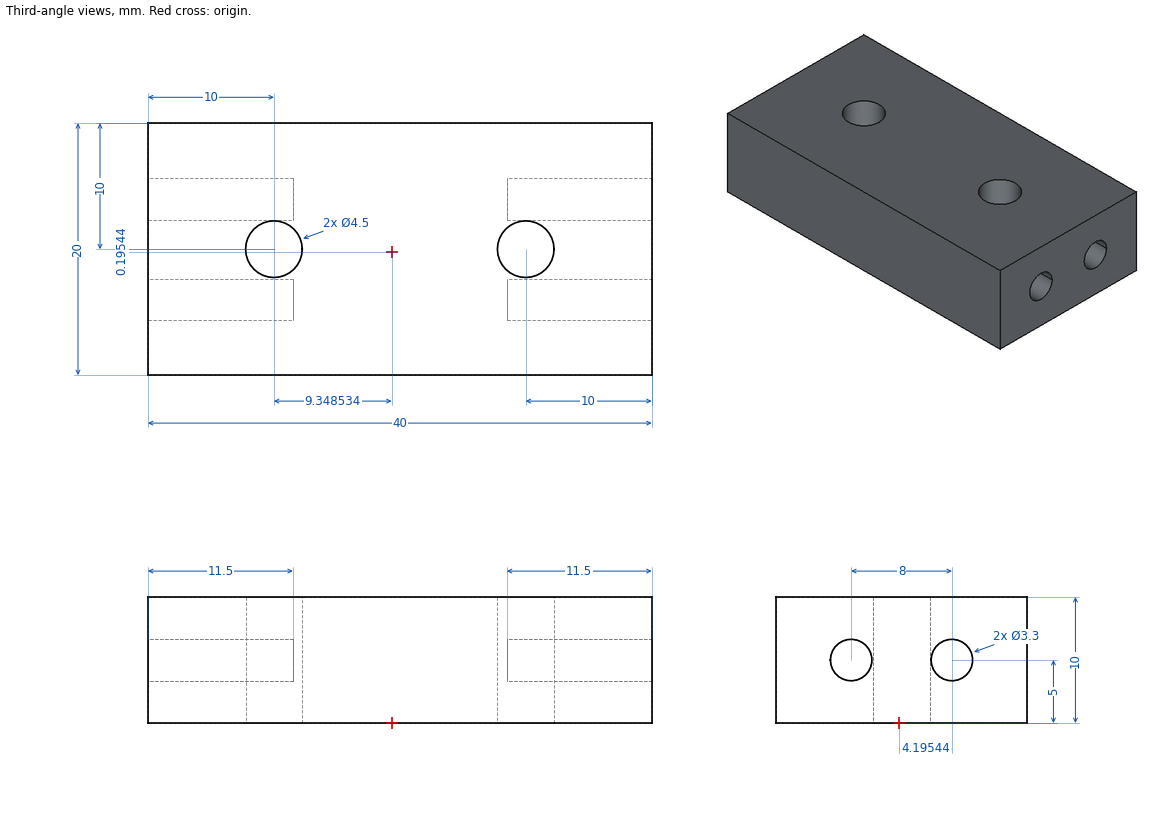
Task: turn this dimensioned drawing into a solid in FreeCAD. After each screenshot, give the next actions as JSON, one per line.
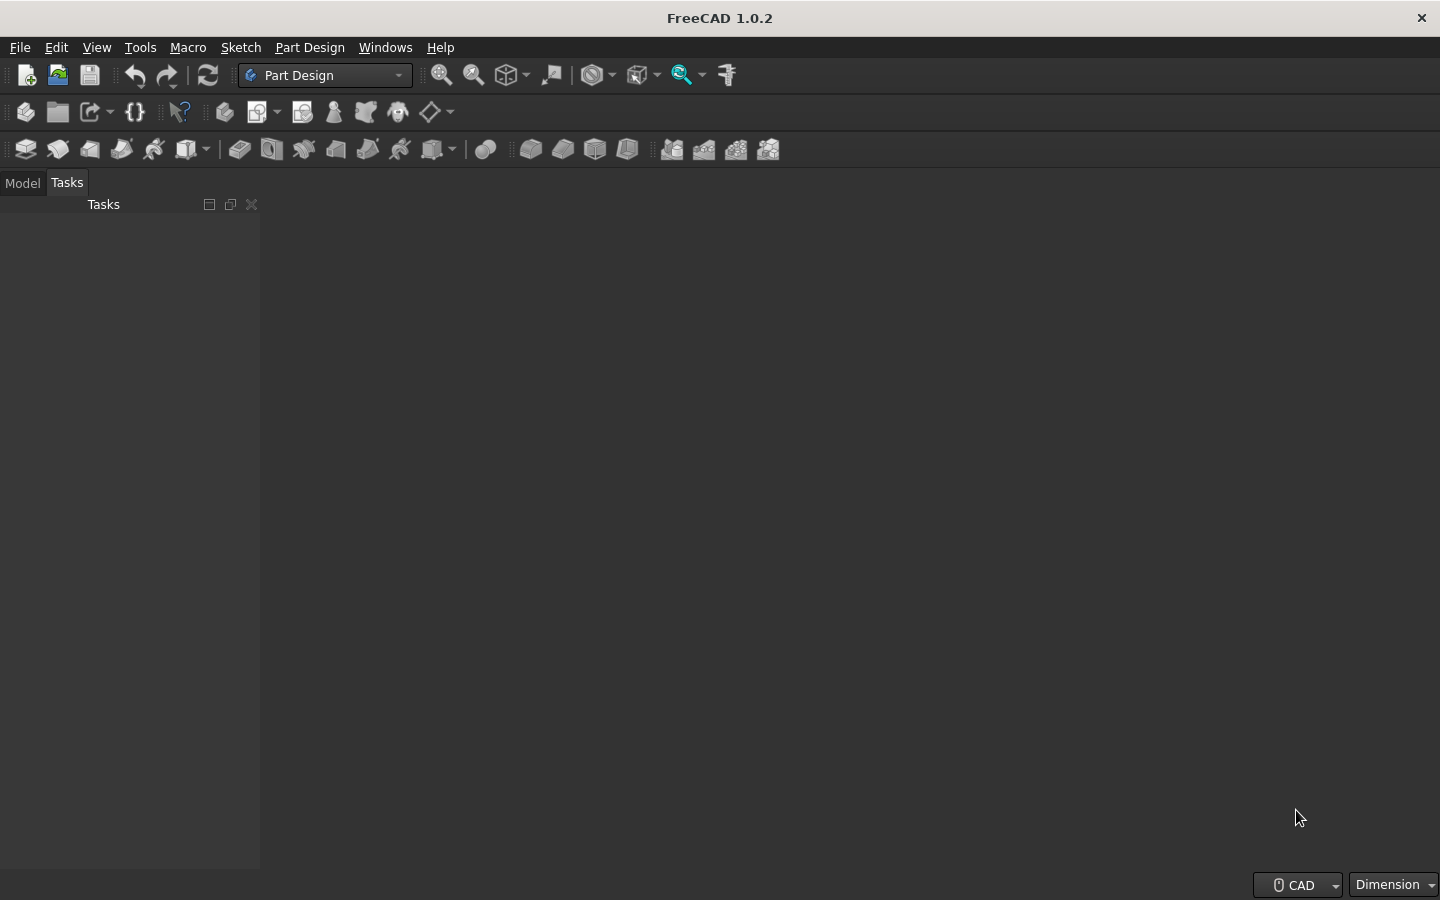
{"action": "left_click", "coordinate": [26, 76]}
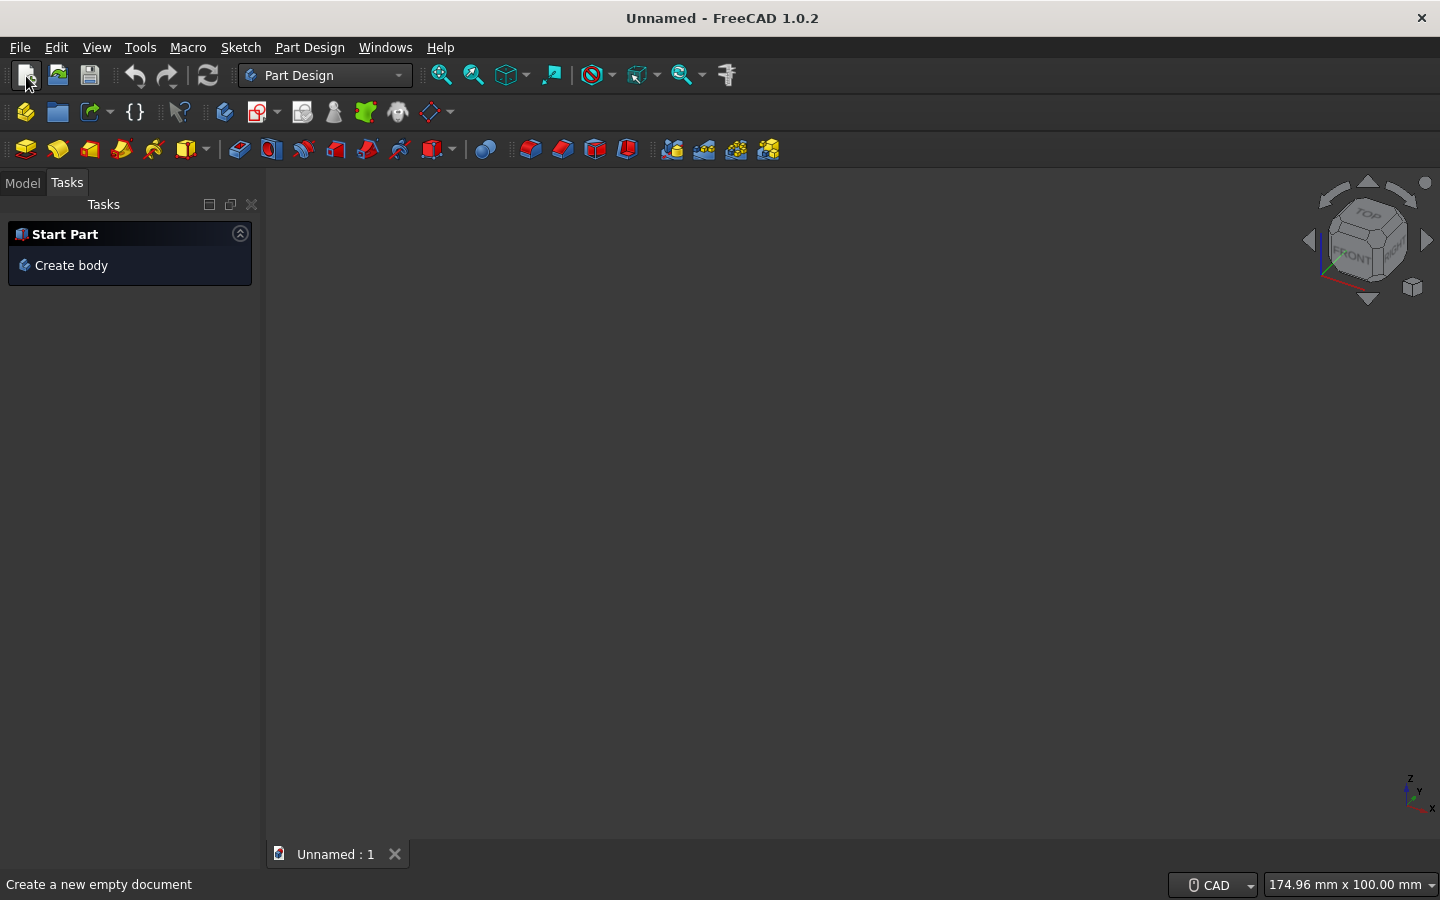
{"action": "left_click", "coordinate": [258, 112]}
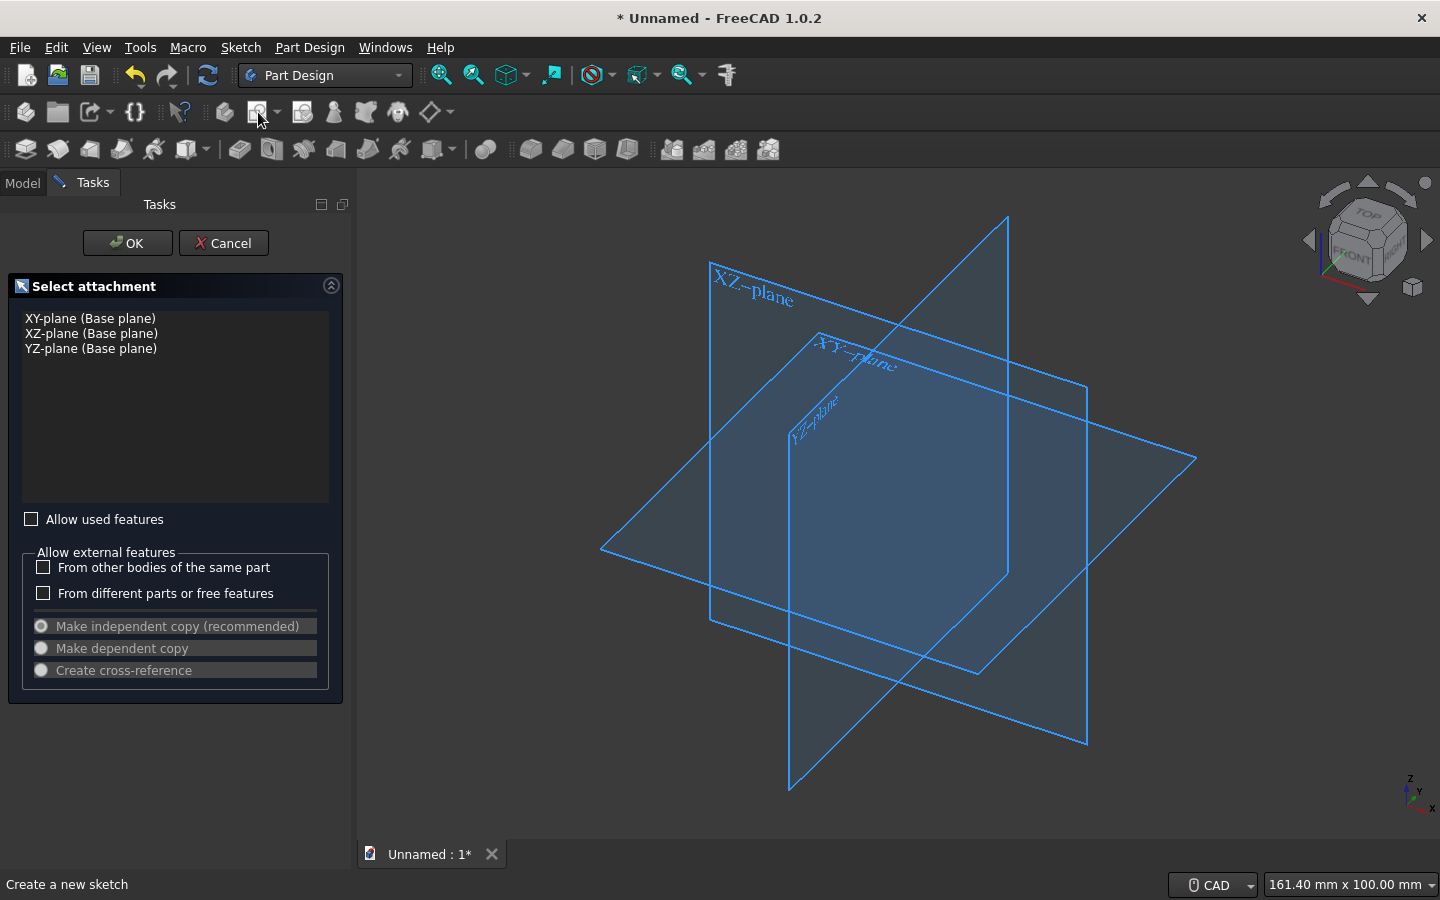
{"action": "left_click", "coordinate": [82, 318]}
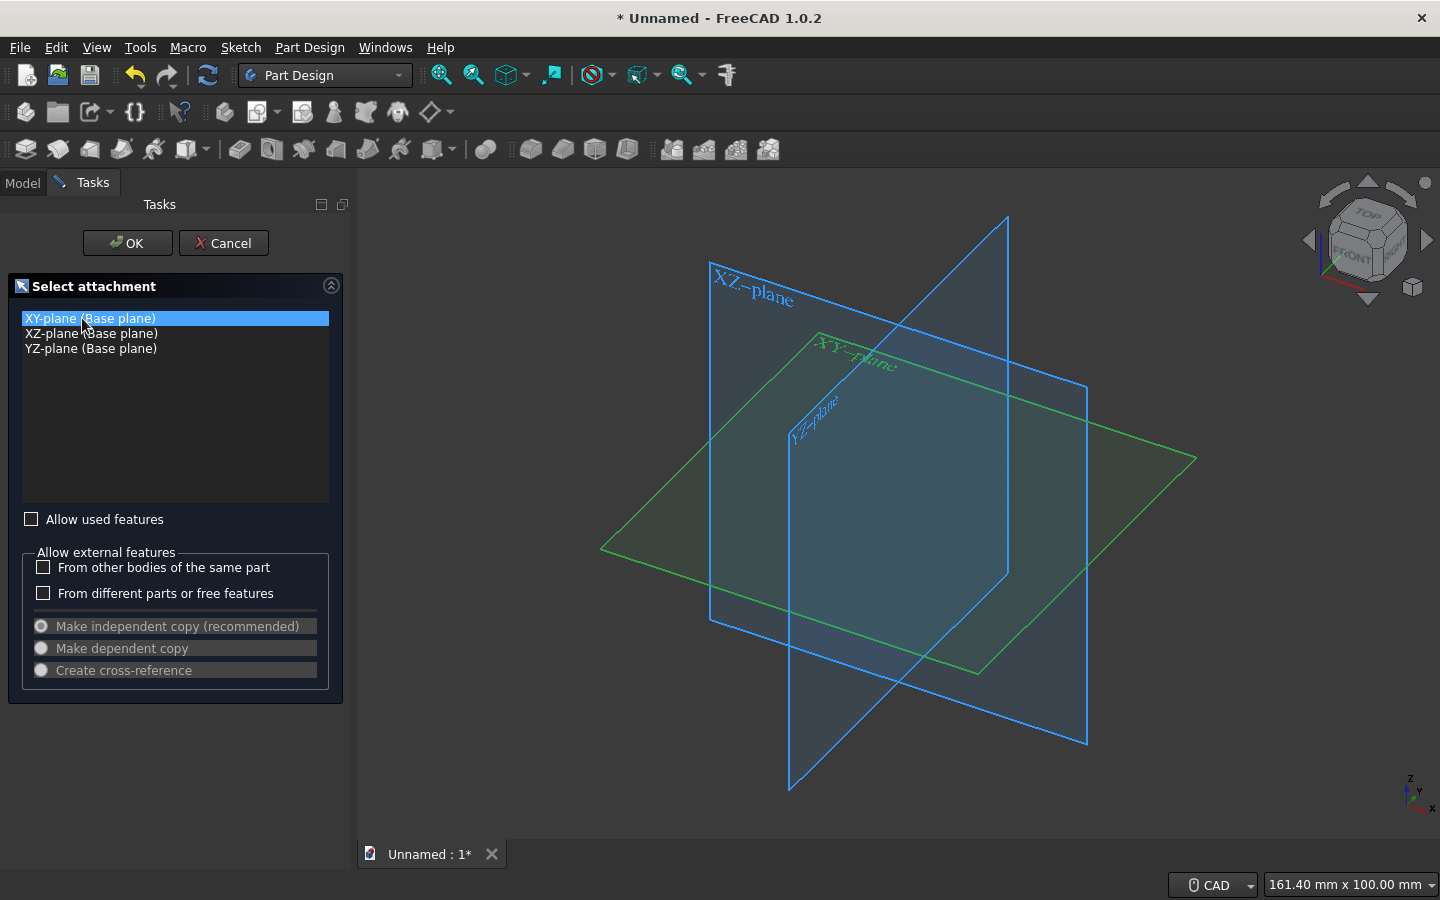
{"action": "left_click", "coordinate": [128, 243]}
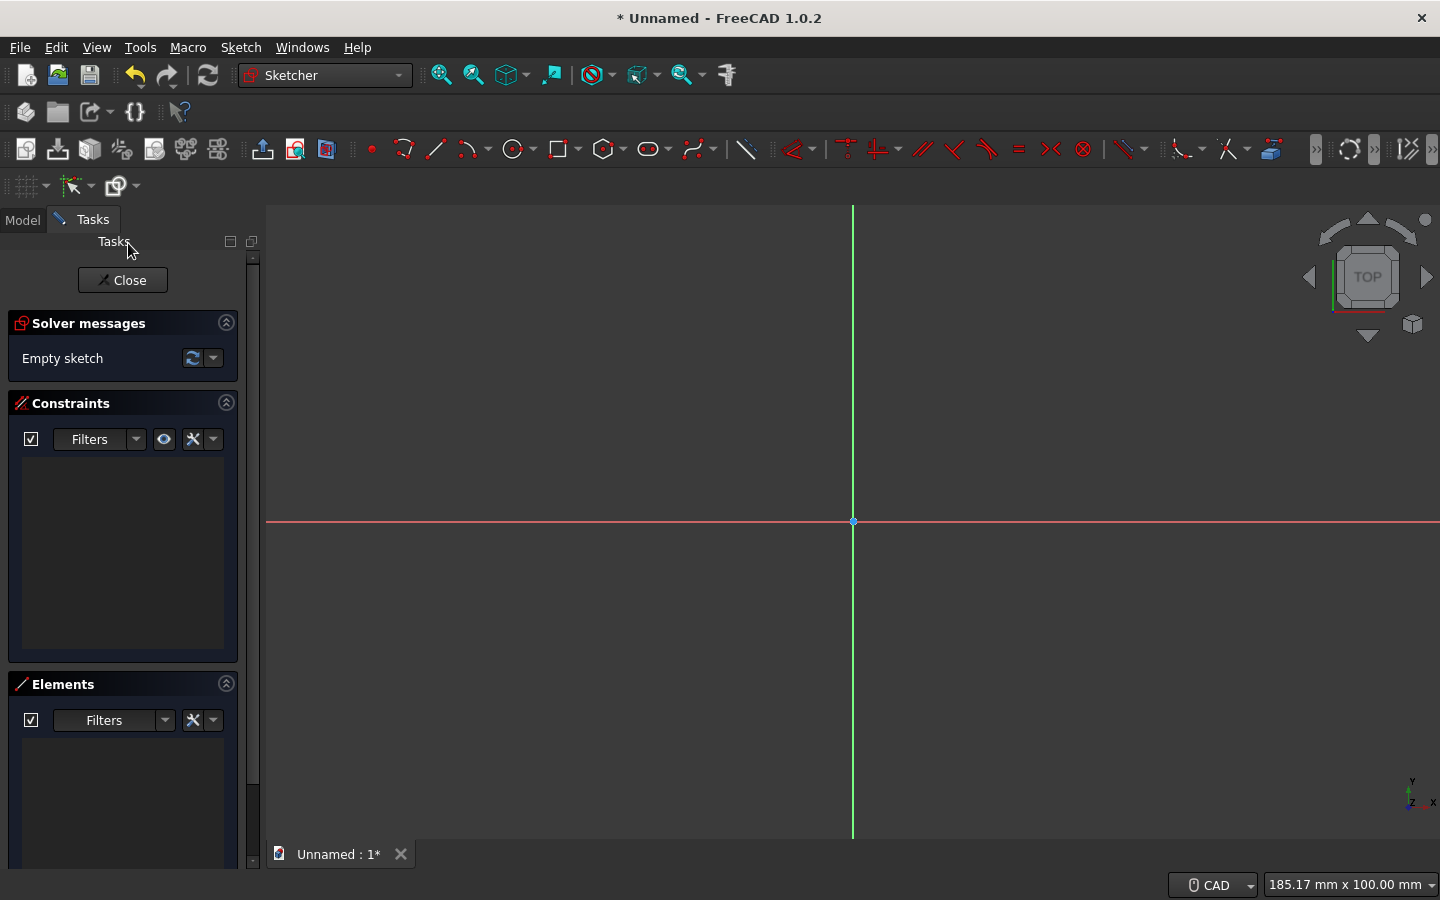
{"action": "scroll", "coordinate": [899, 520], "scroll_direction": "up", "scroll_amount": 5}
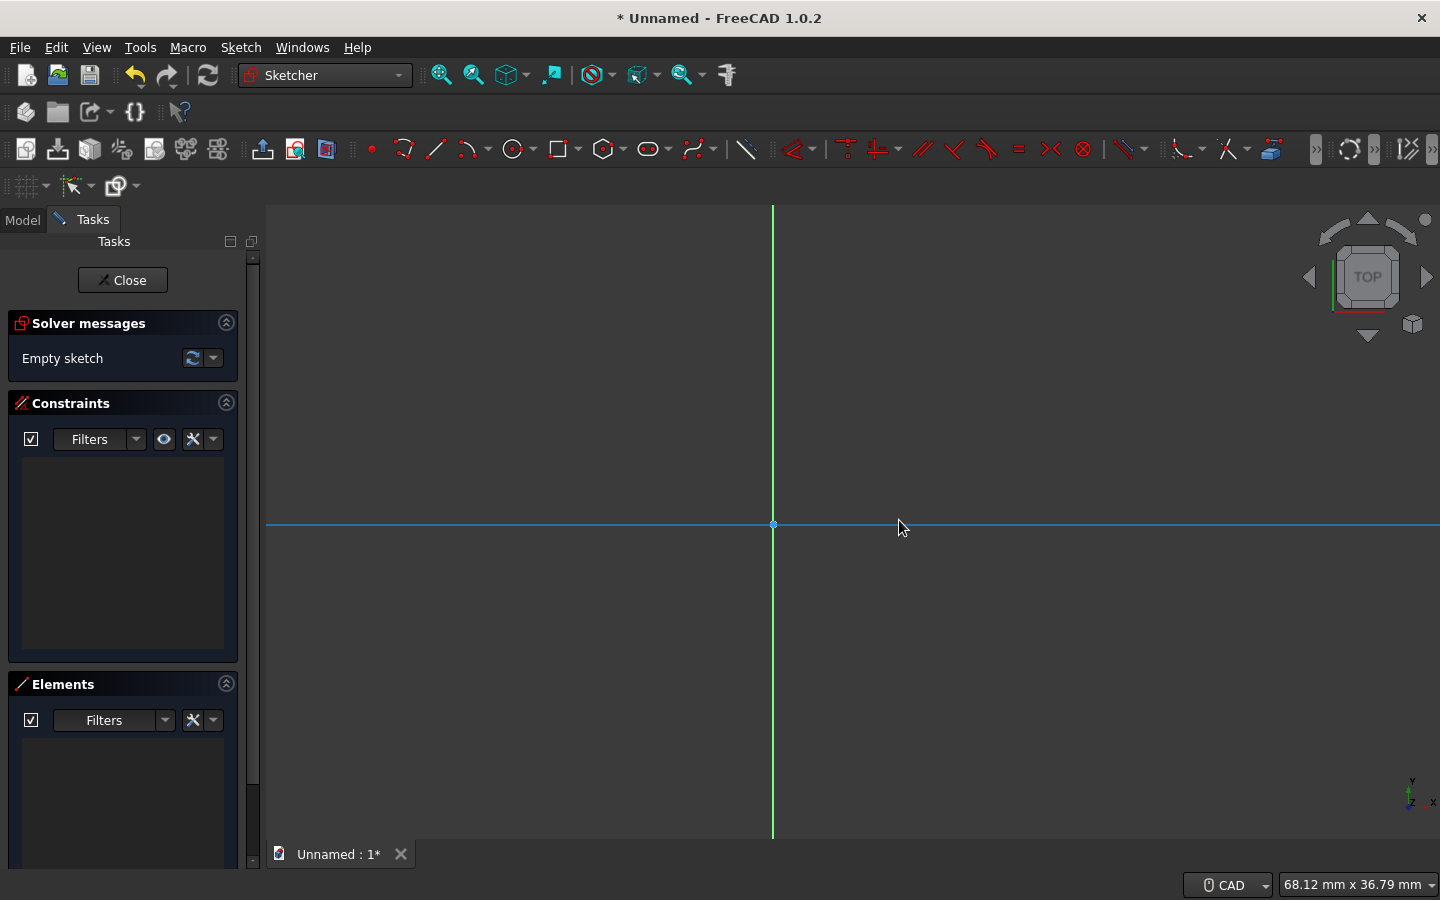
{"action": "key", "text": "g r"}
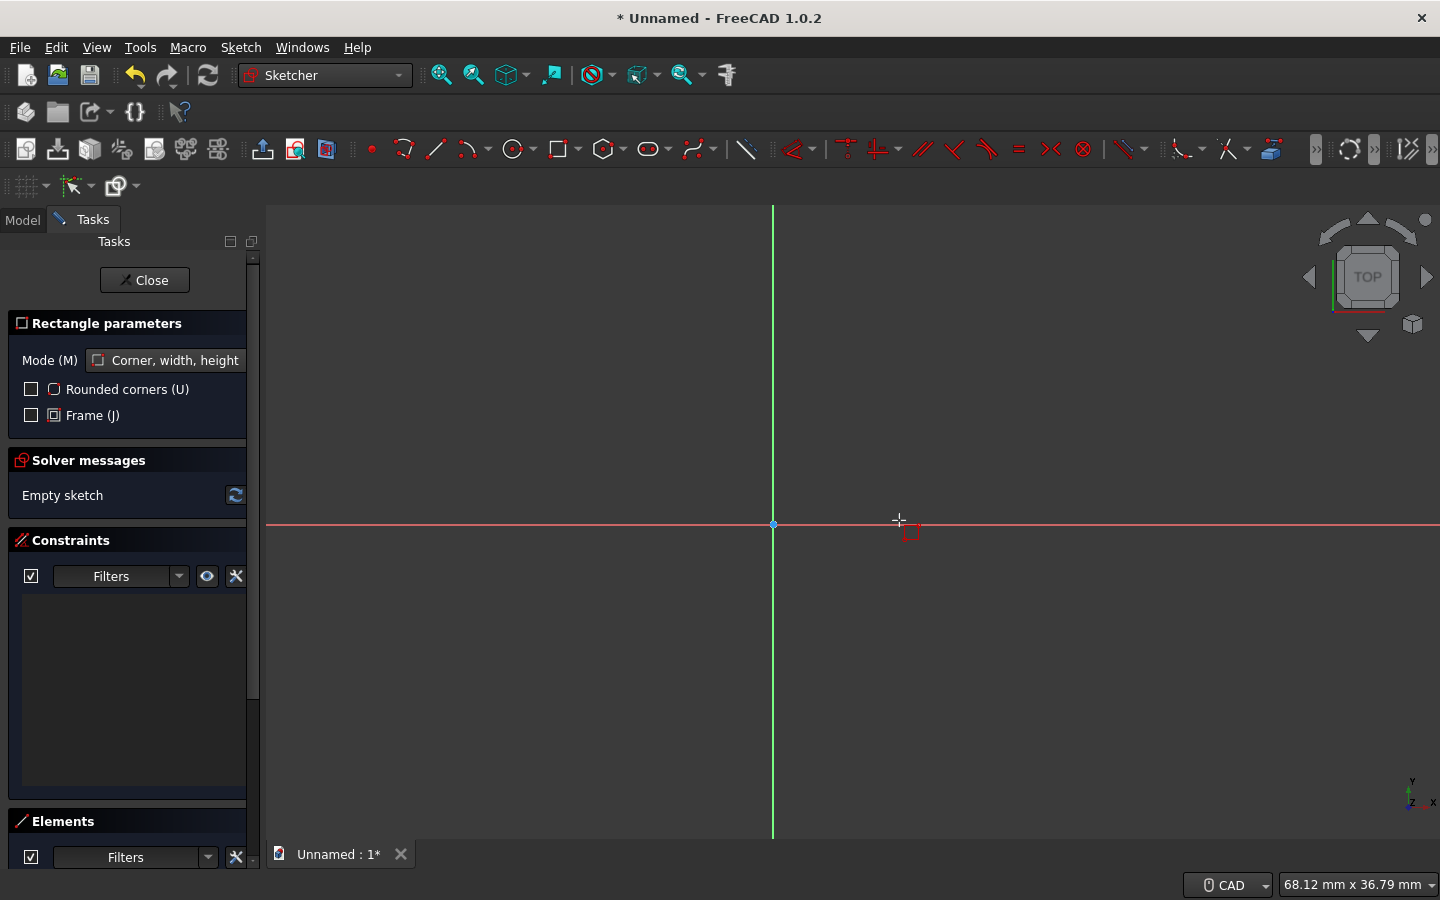
{"action": "left_click", "coordinate": [440, 349]}
{"action": "left_click", "coordinate": [1129, 694]}